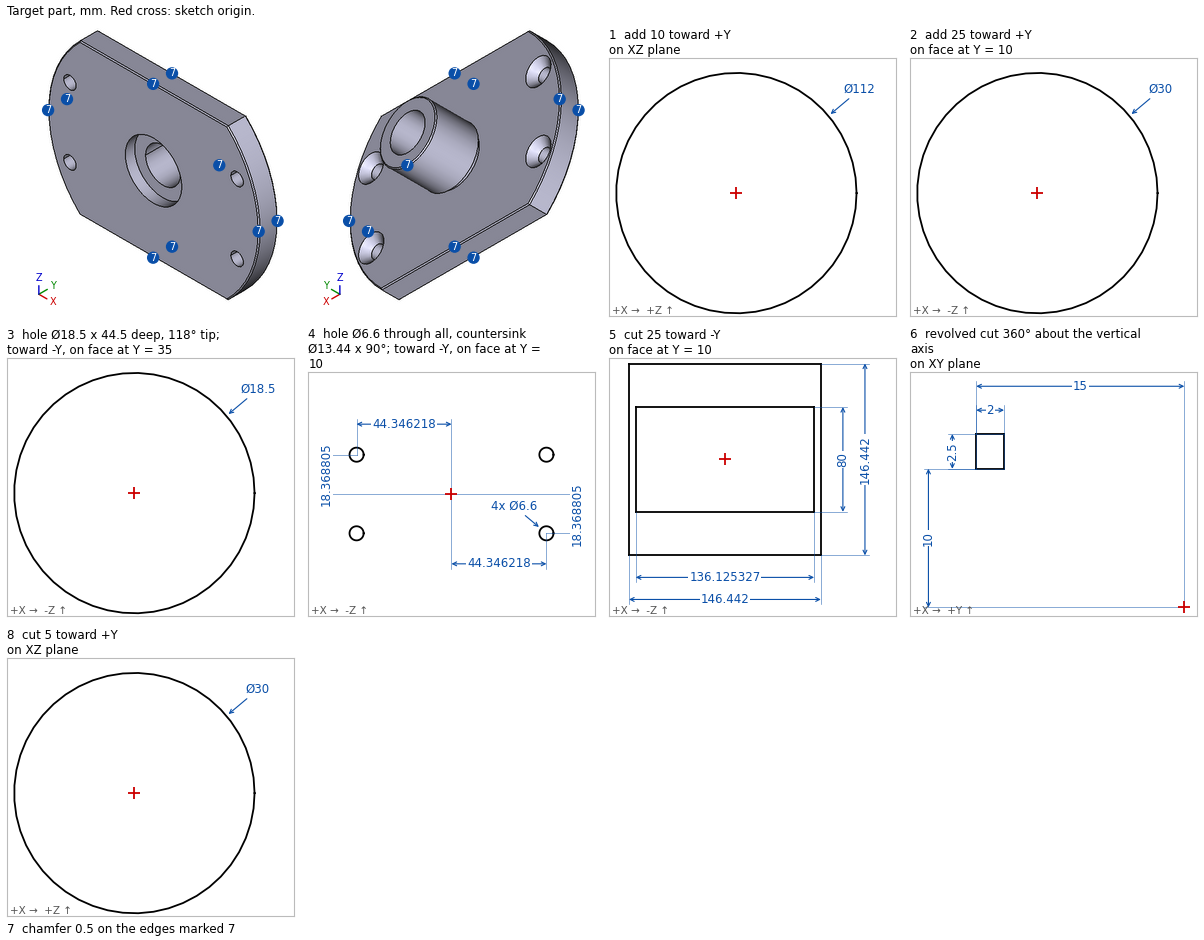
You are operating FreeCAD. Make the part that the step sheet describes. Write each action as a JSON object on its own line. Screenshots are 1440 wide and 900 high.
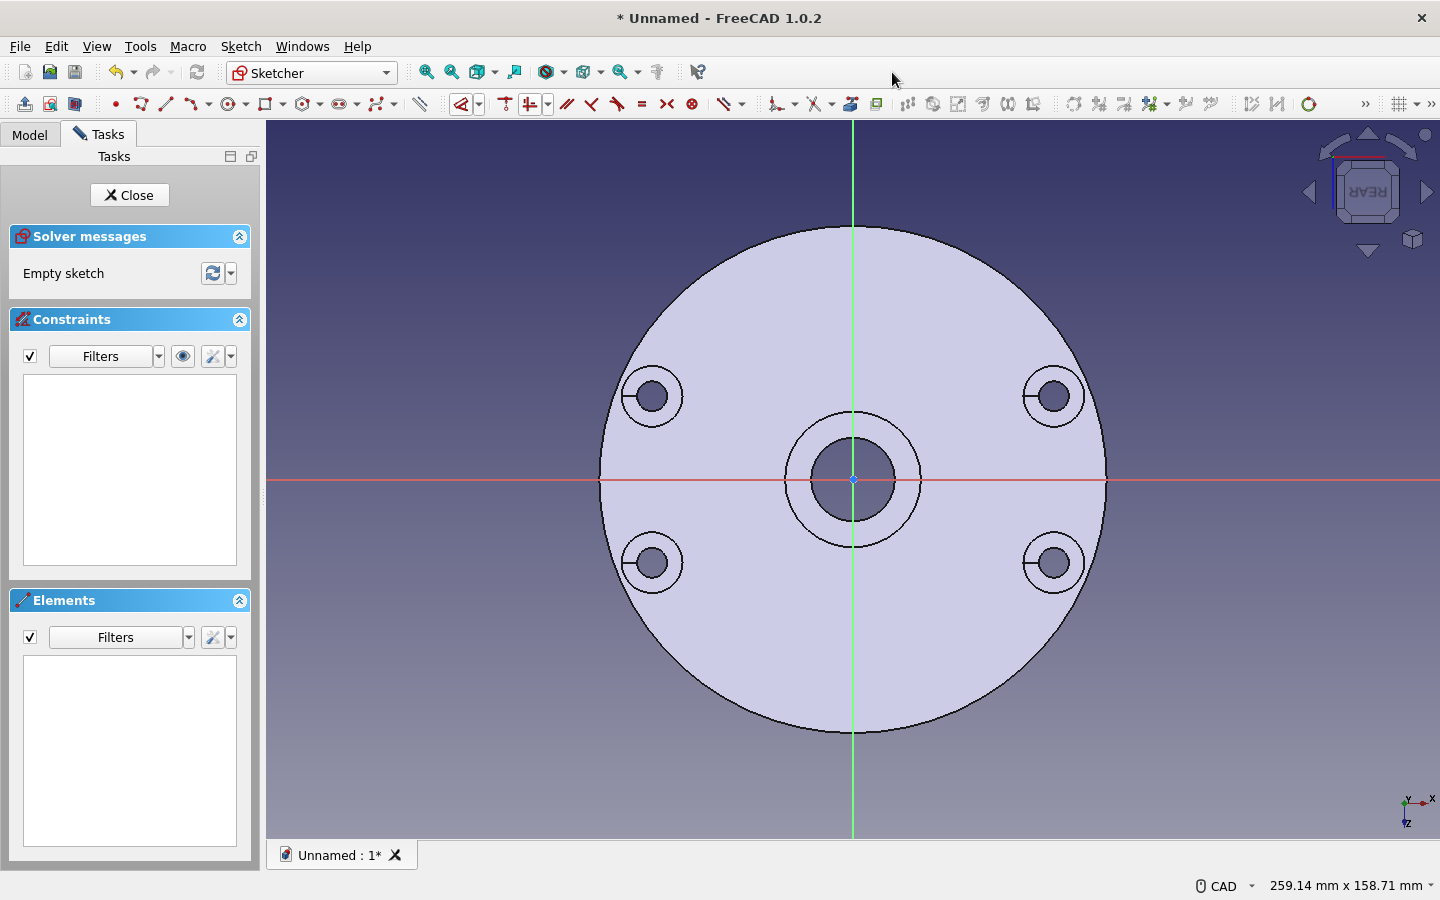
{"action": "scroll", "coordinate": [645, 480], "scroll_direction": "down", "scroll_amount": 2}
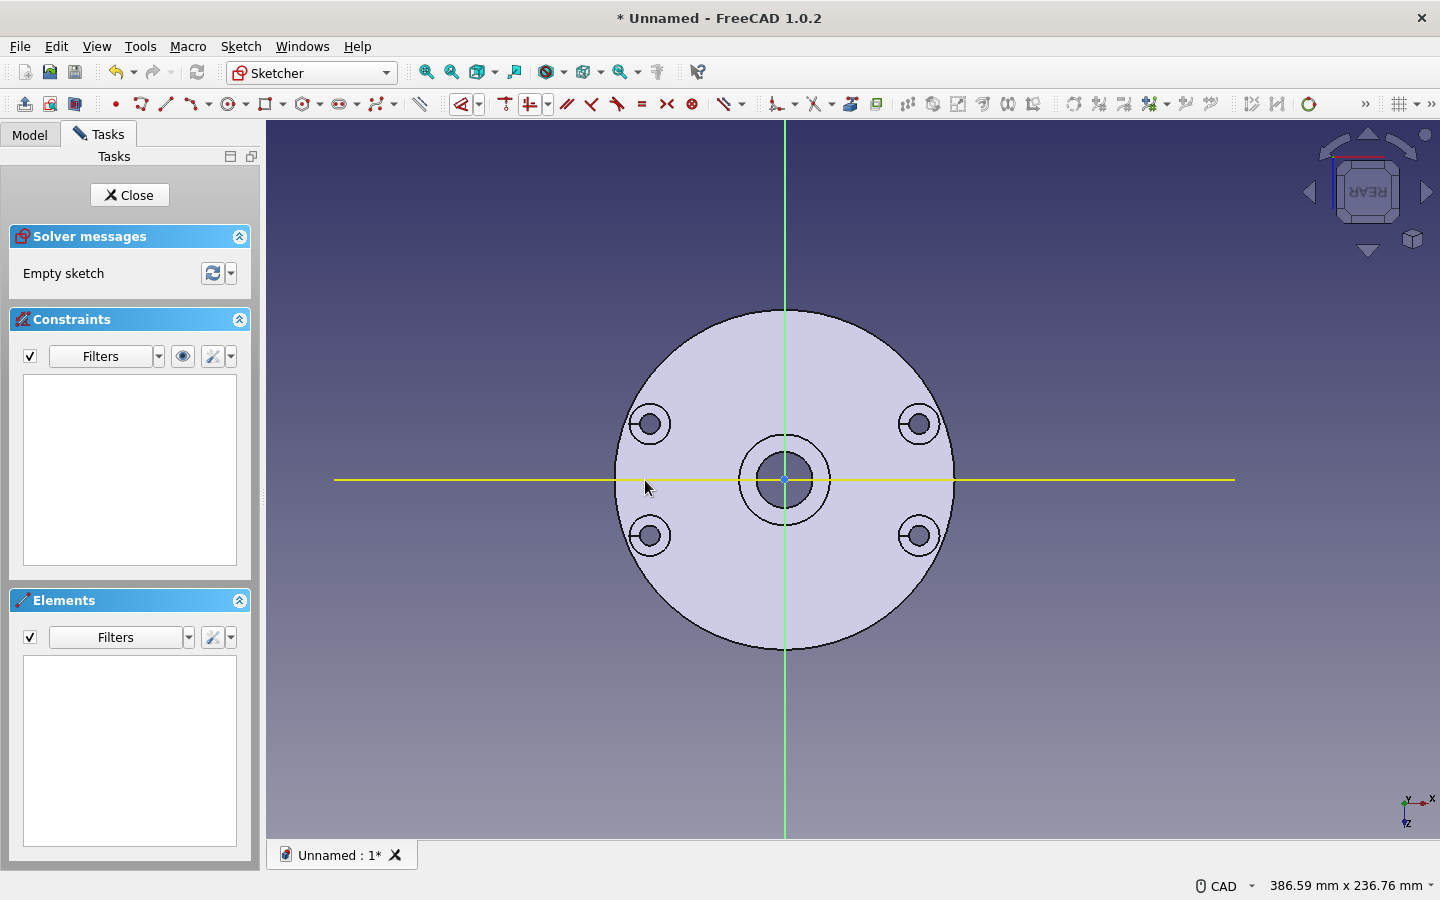
{"action": "key", "text": "g v"}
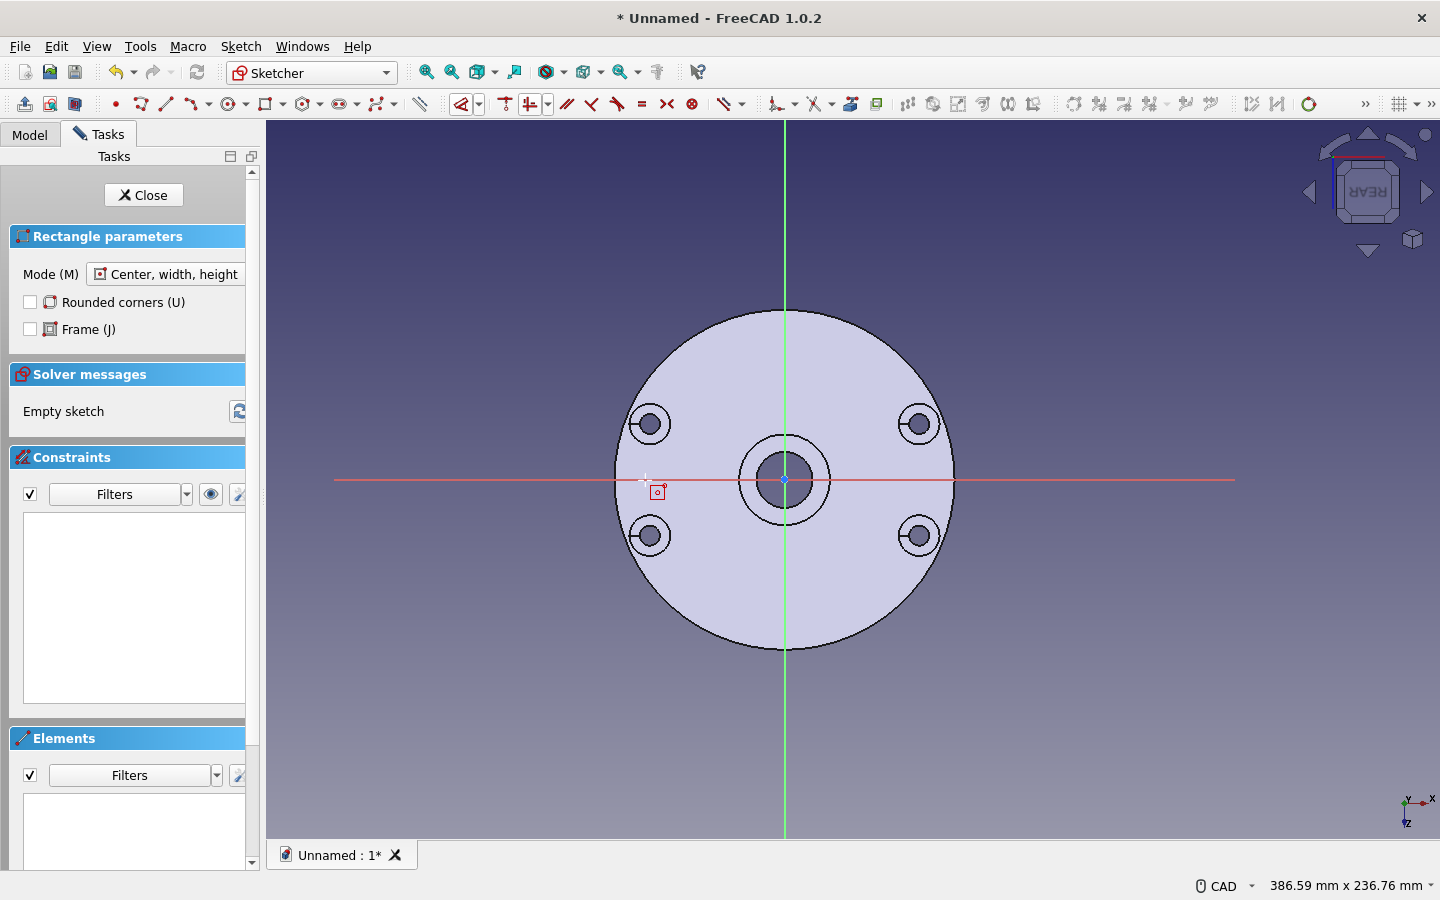
{"action": "left_click", "coordinate": [785, 480]}
{"action": "mouse_move", "coordinate": [1007, 257]}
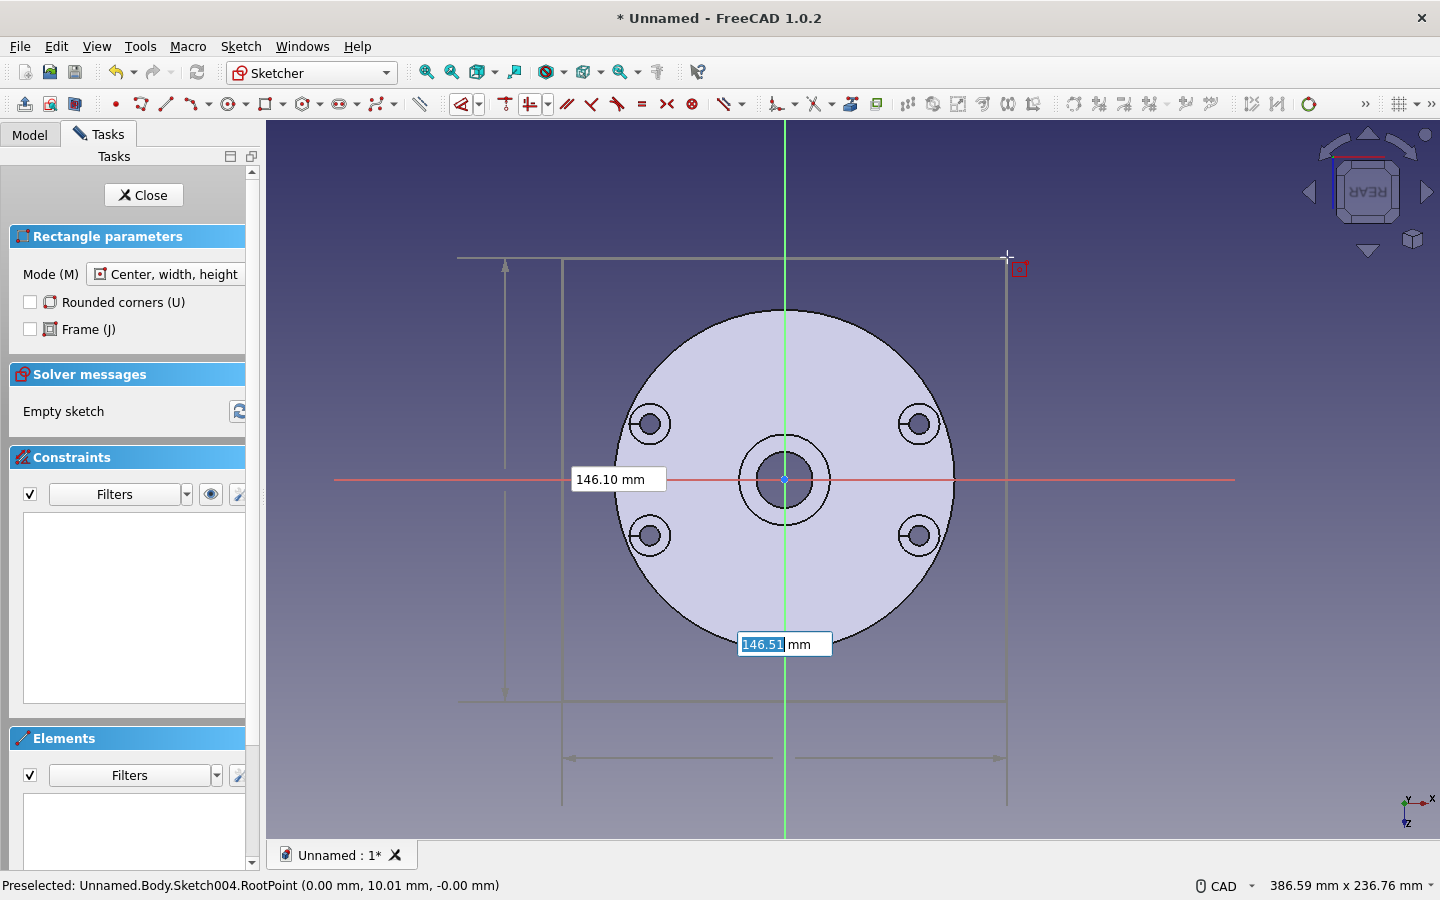
{"action": "type", "text": "146.442"}
{"action": "key", "text": "Tab"}
{"action": "type", "text": "146.442"}
{"action": "key", "text": "Return"}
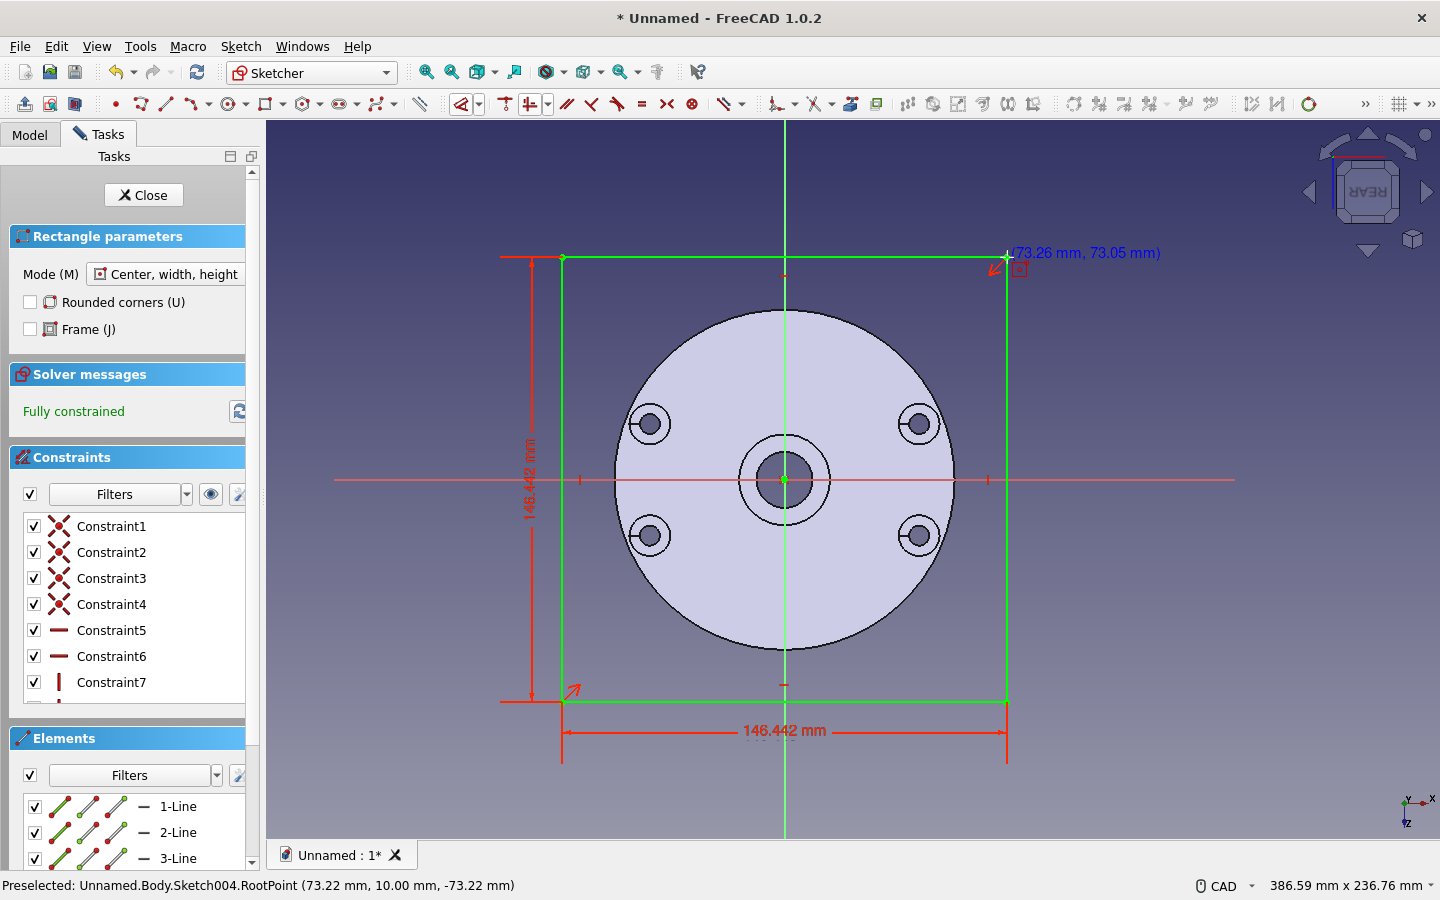
{"action": "left_click", "coordinate": [785, 480]}
{"action": "mouse_move", "coordinate": [991, 358]}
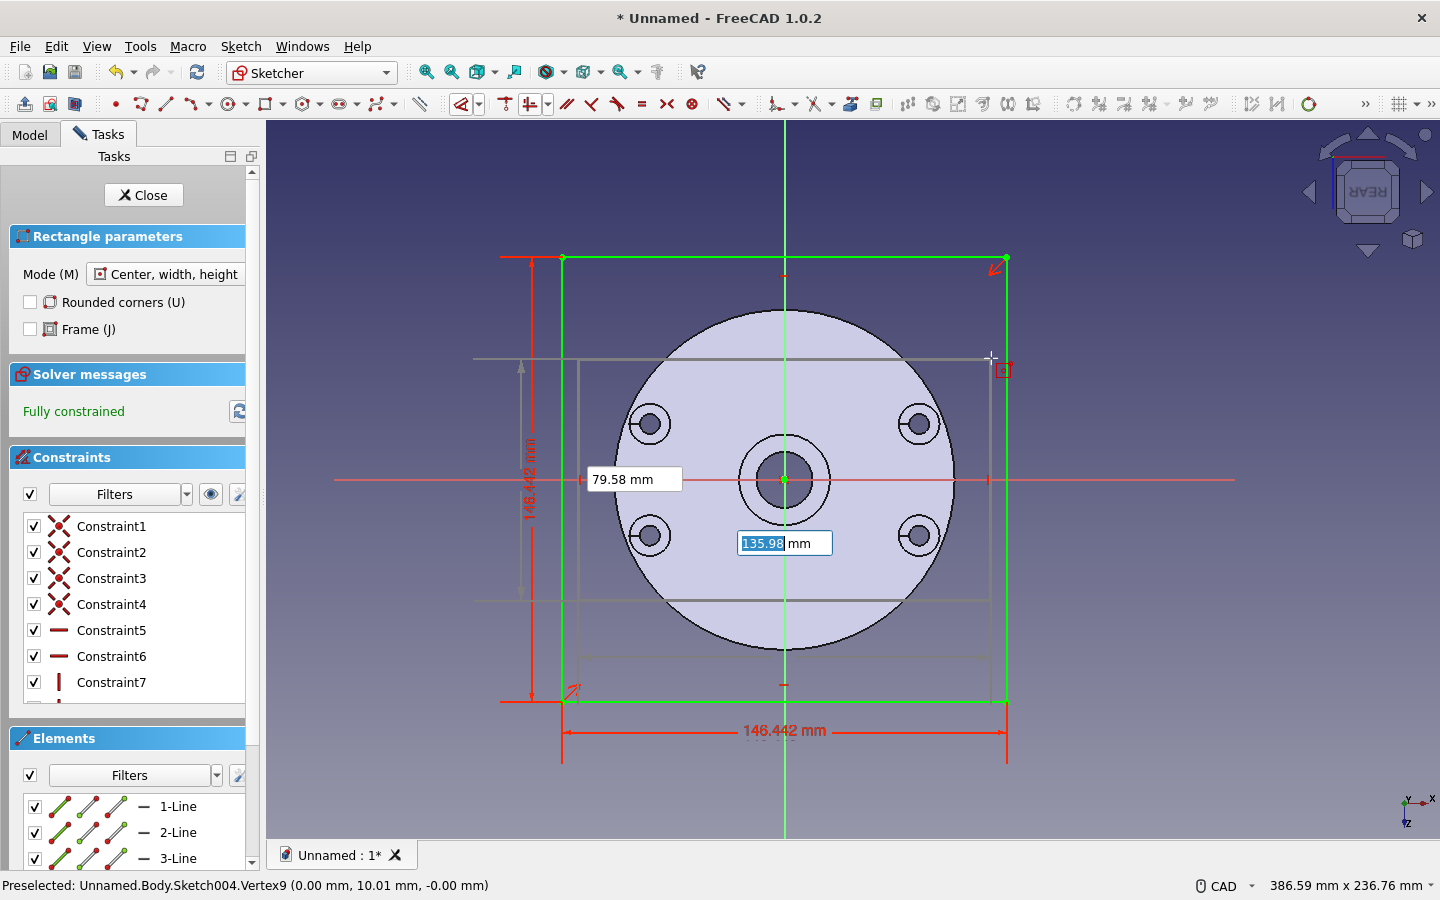
{"action": "type", "text": "136.125327"}
{"action": "key", "text": "Tab"}
{"action": "type", "text": "80"}
{"action": "key", "text": "Return"}
{"action": "key", "text": "Escape"}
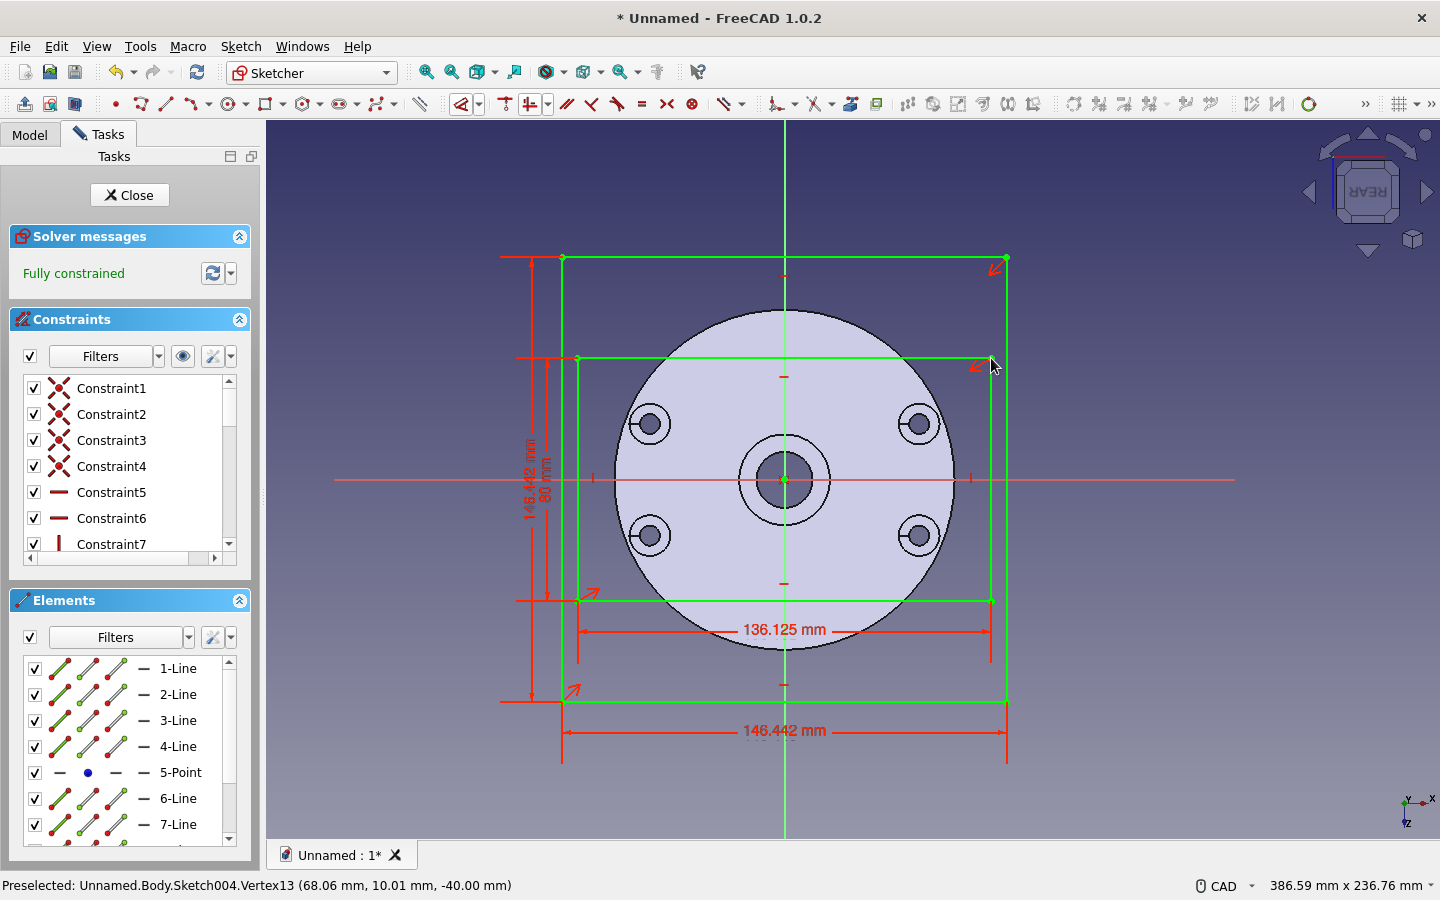
{"action": "left_click", "coordinate": [130, 195]}